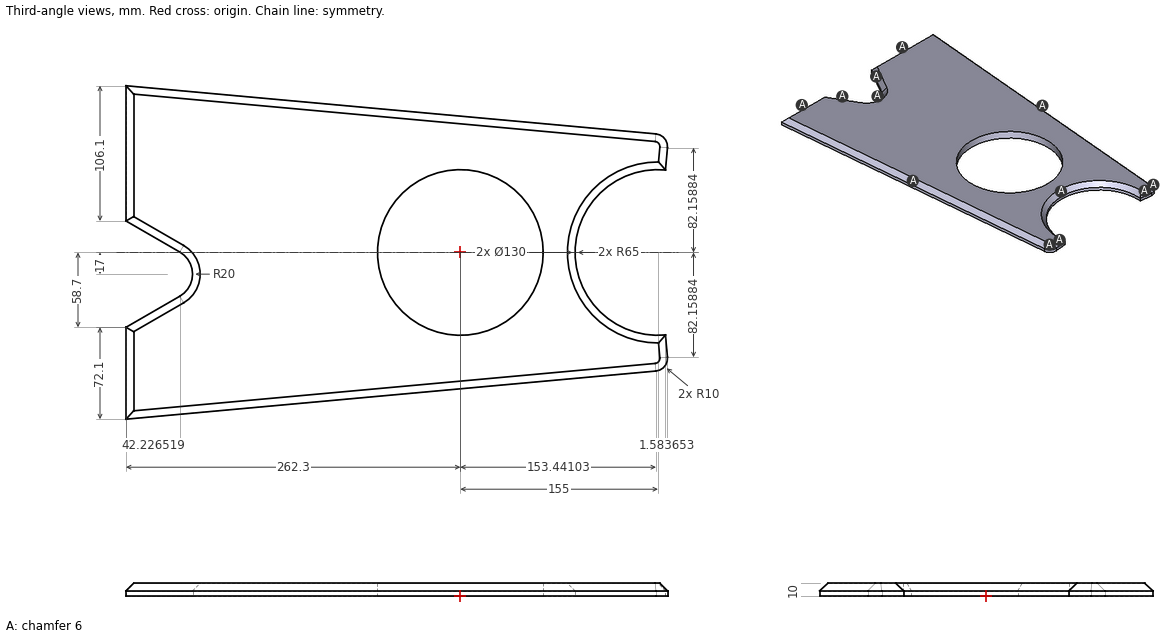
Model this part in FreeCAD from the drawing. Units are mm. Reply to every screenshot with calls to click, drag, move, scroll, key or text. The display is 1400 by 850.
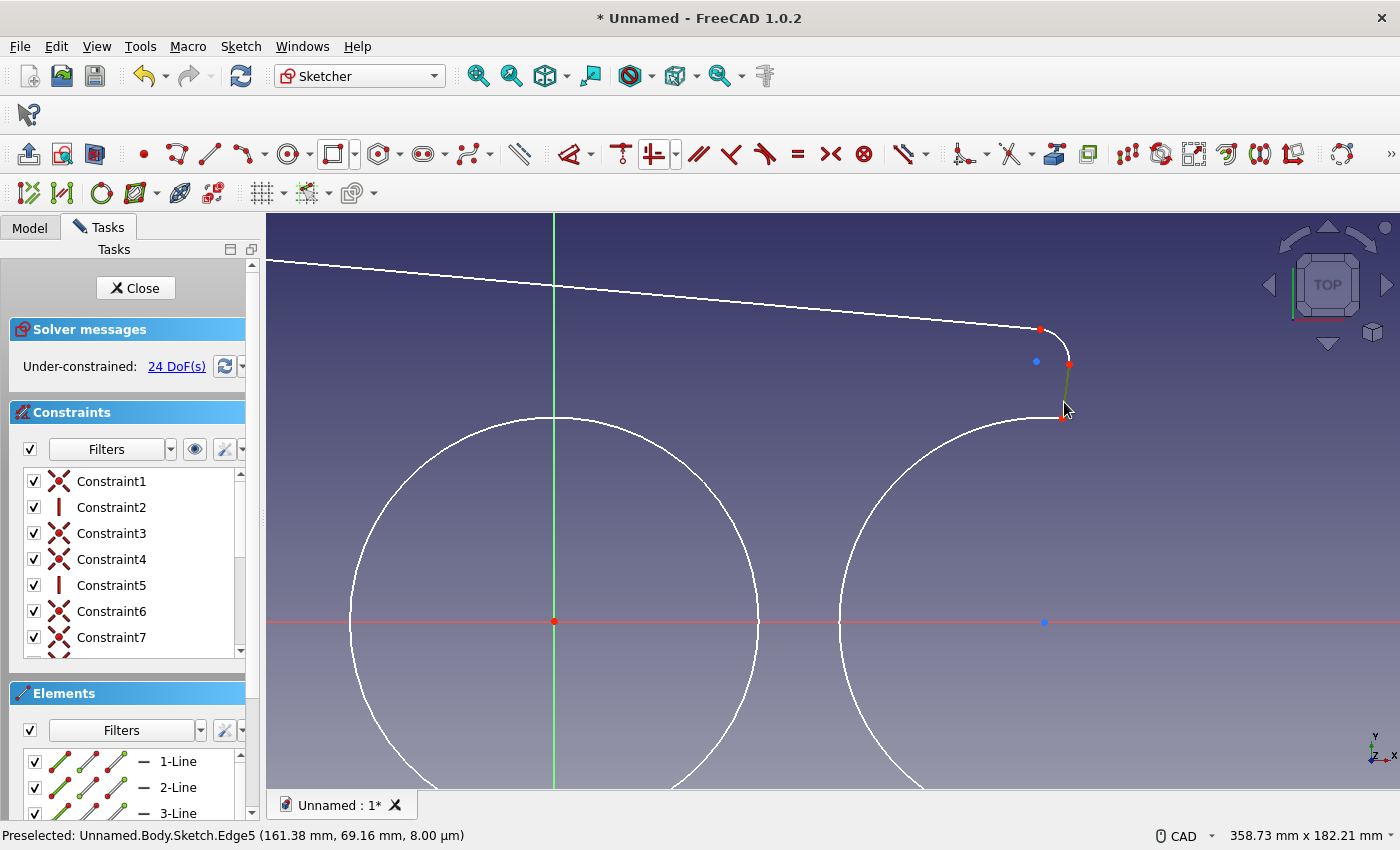
click(1067, 350)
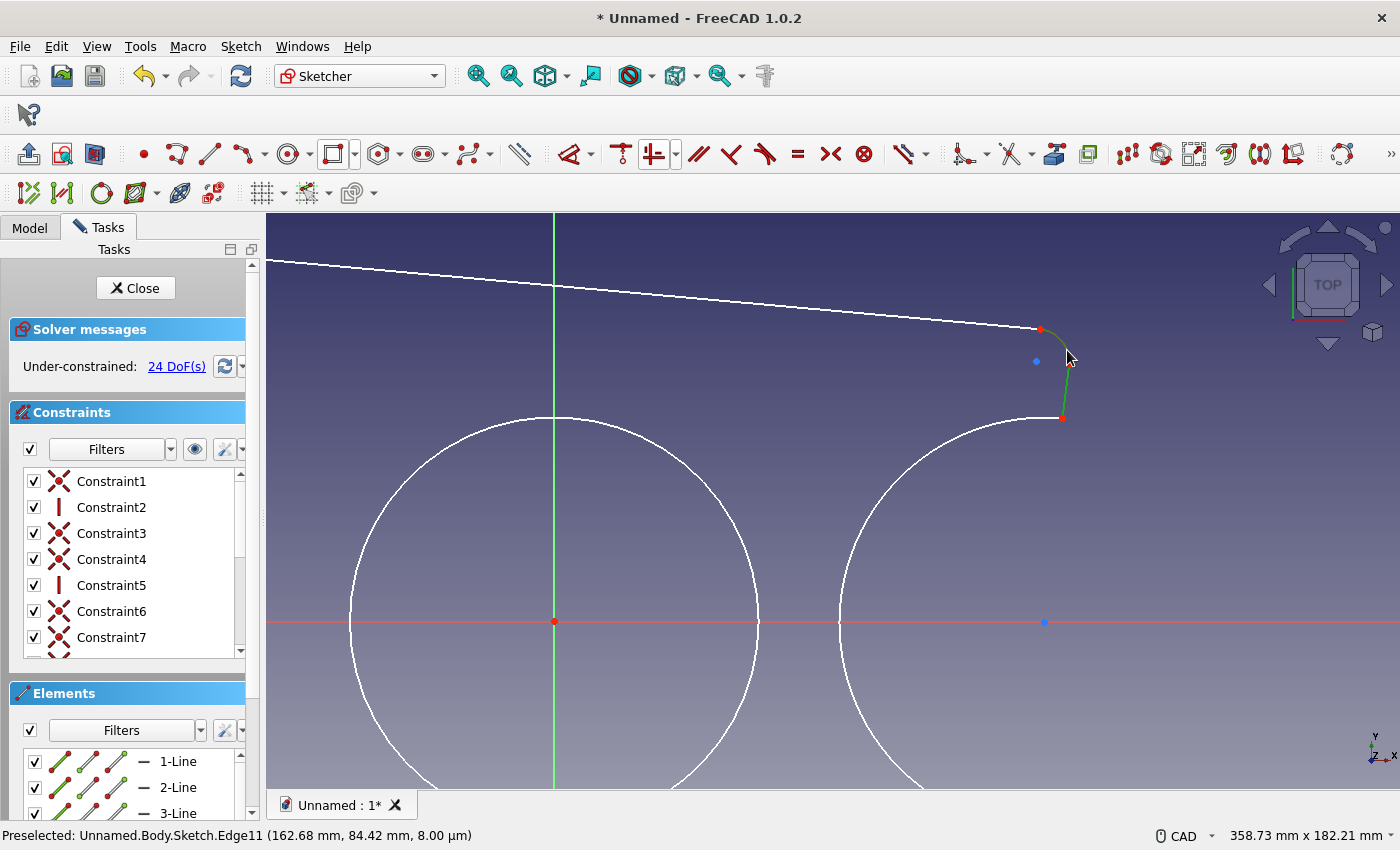
click(765, 154)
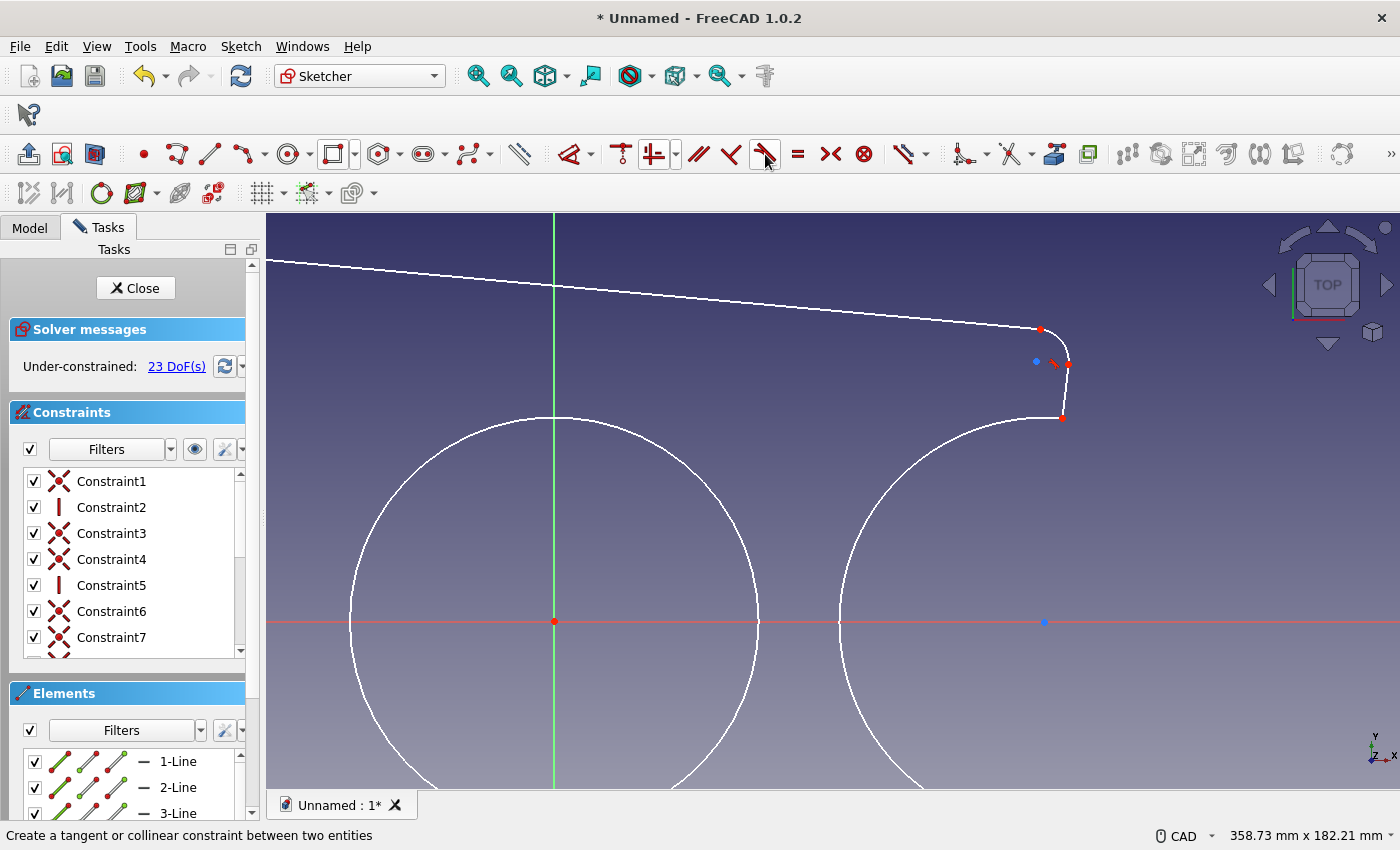
click(646, 294)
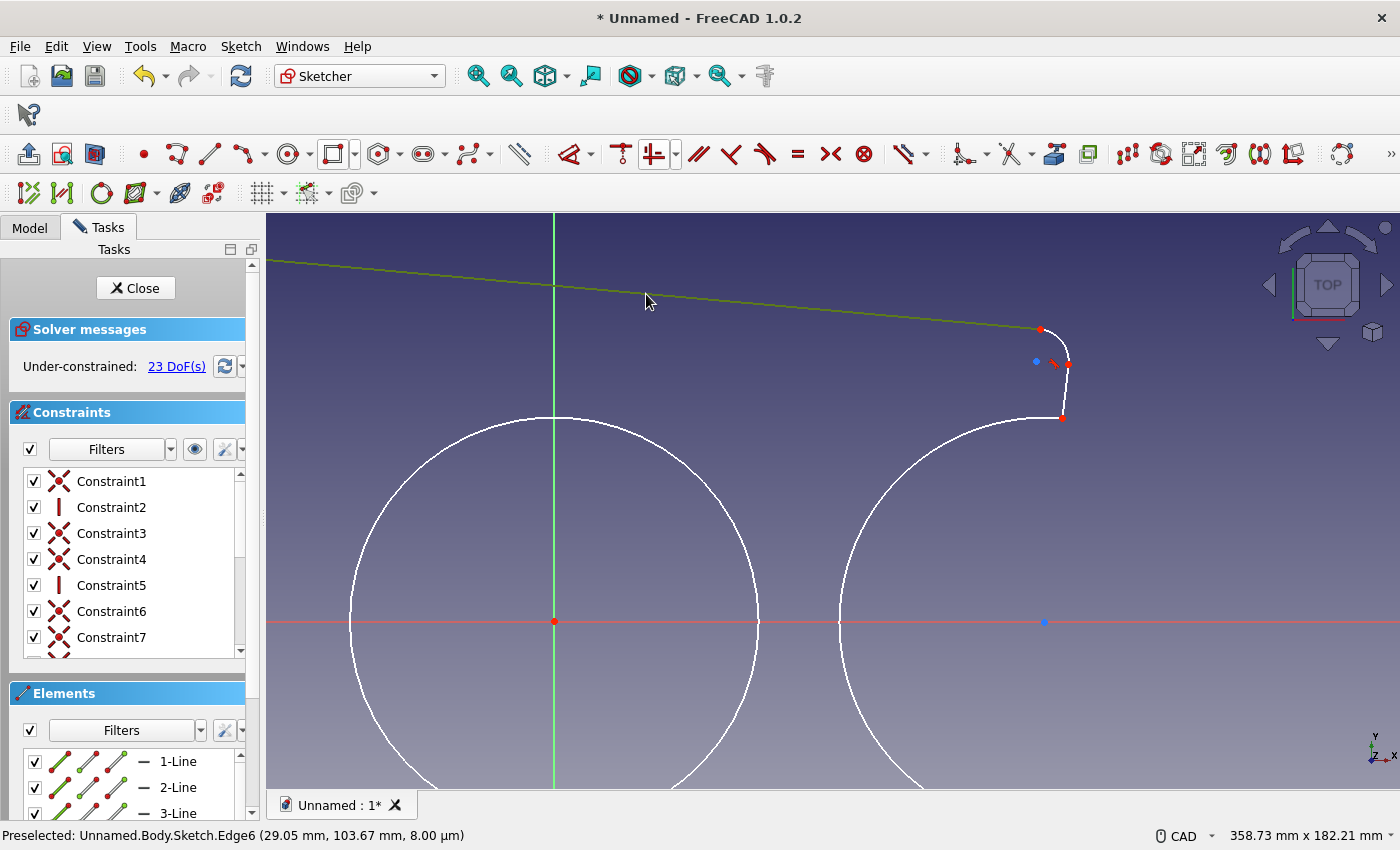
click(1067, 350)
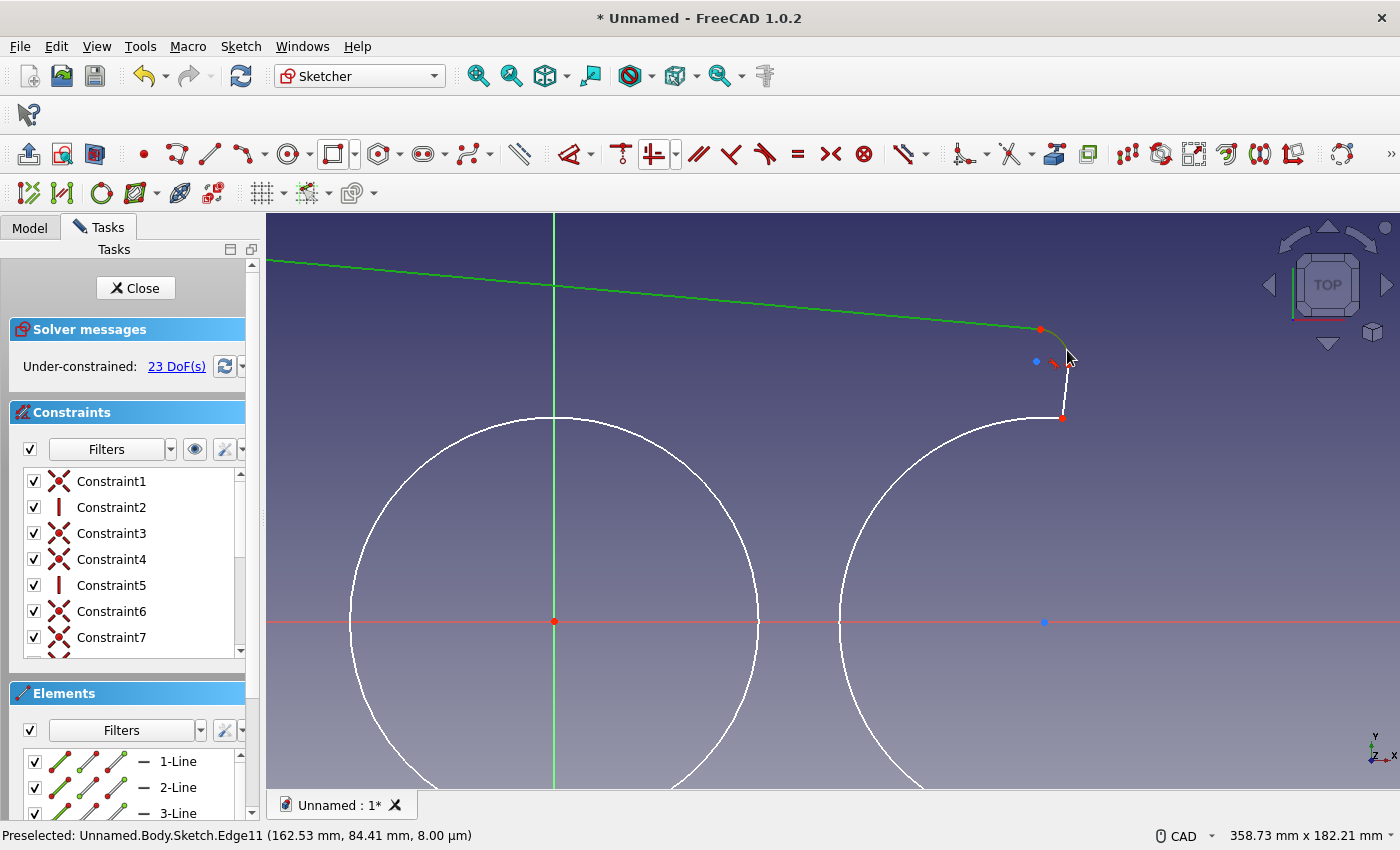
click(765, 154)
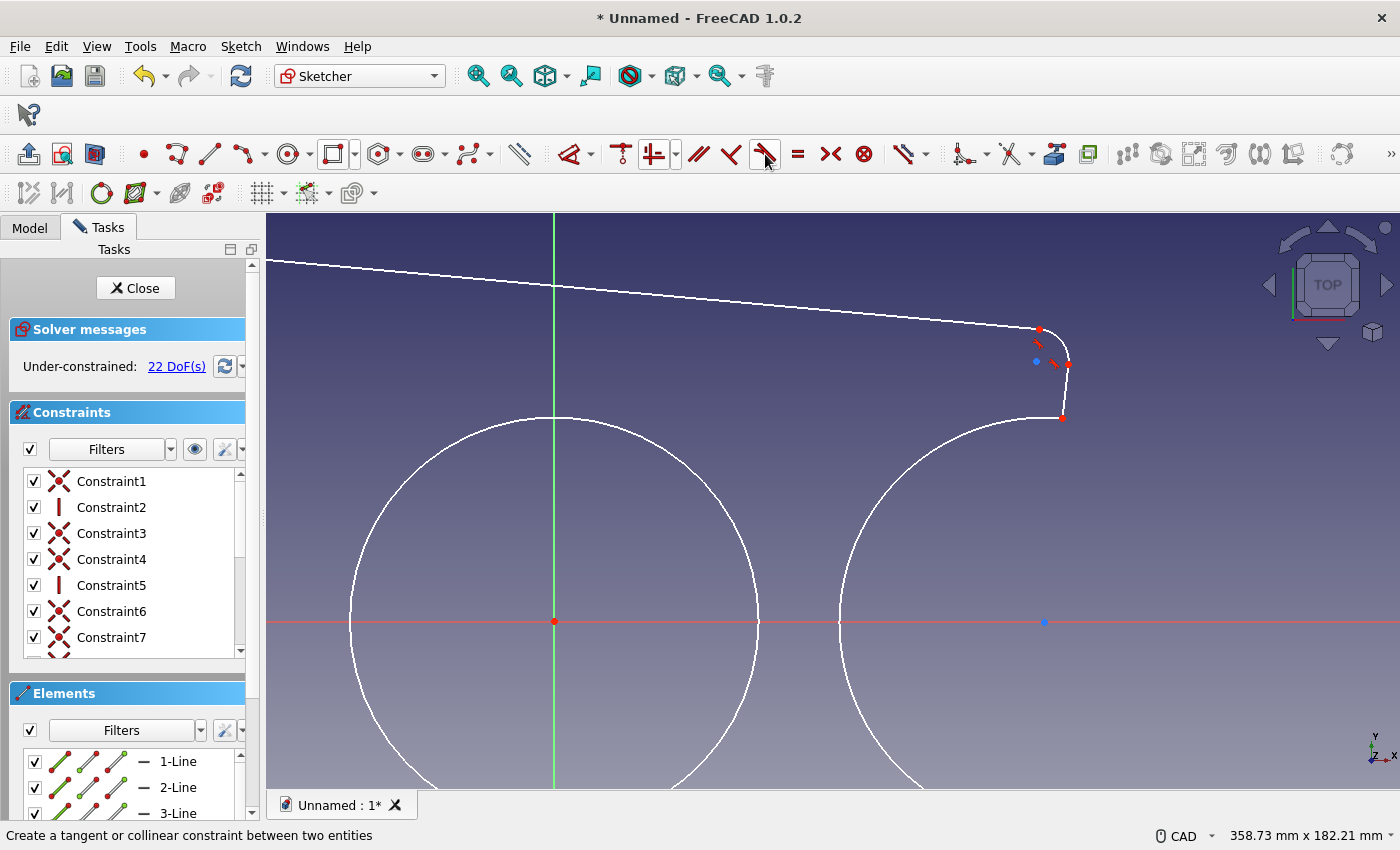
scroll(1065, 403, down, 4)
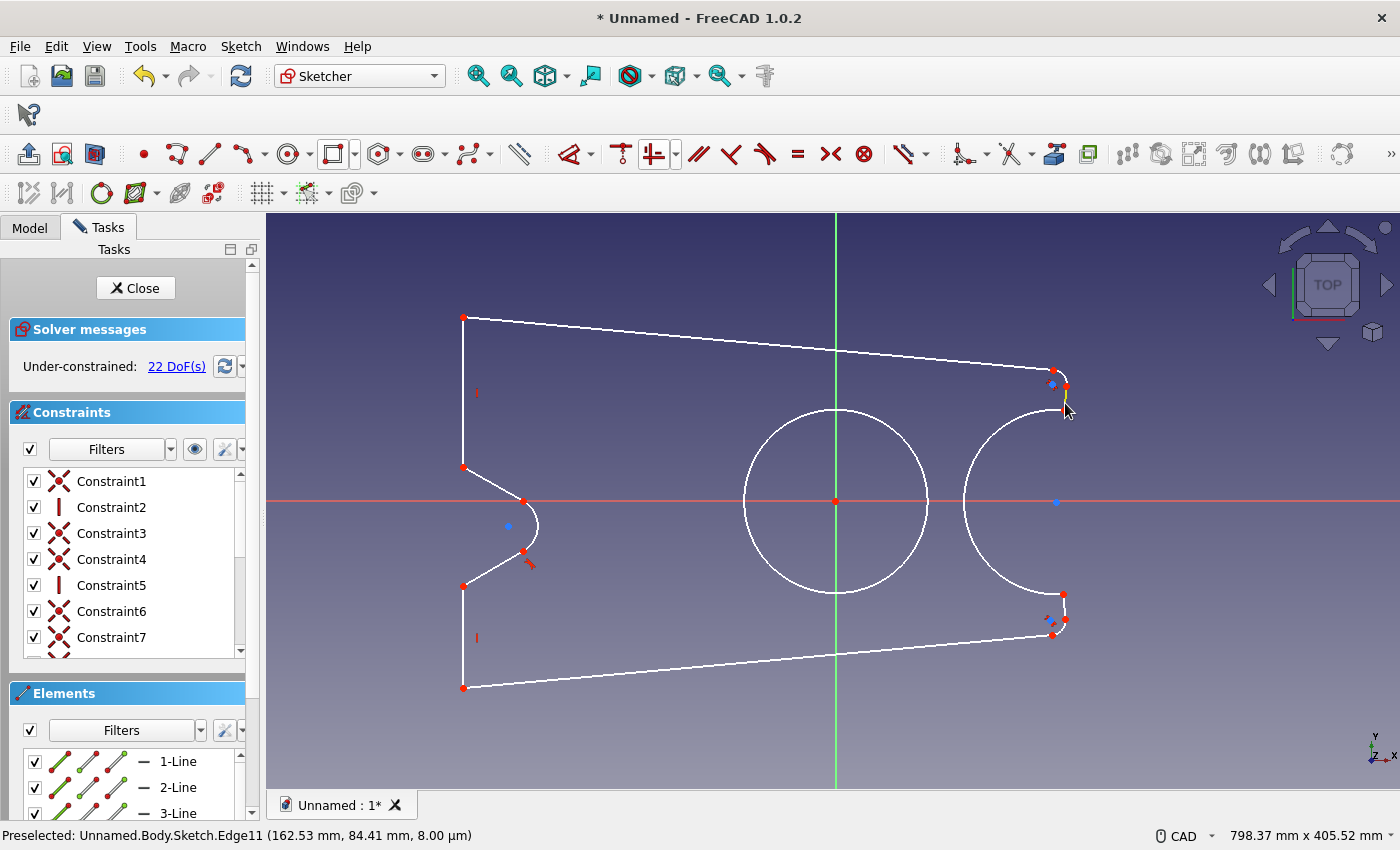
click(481, 477)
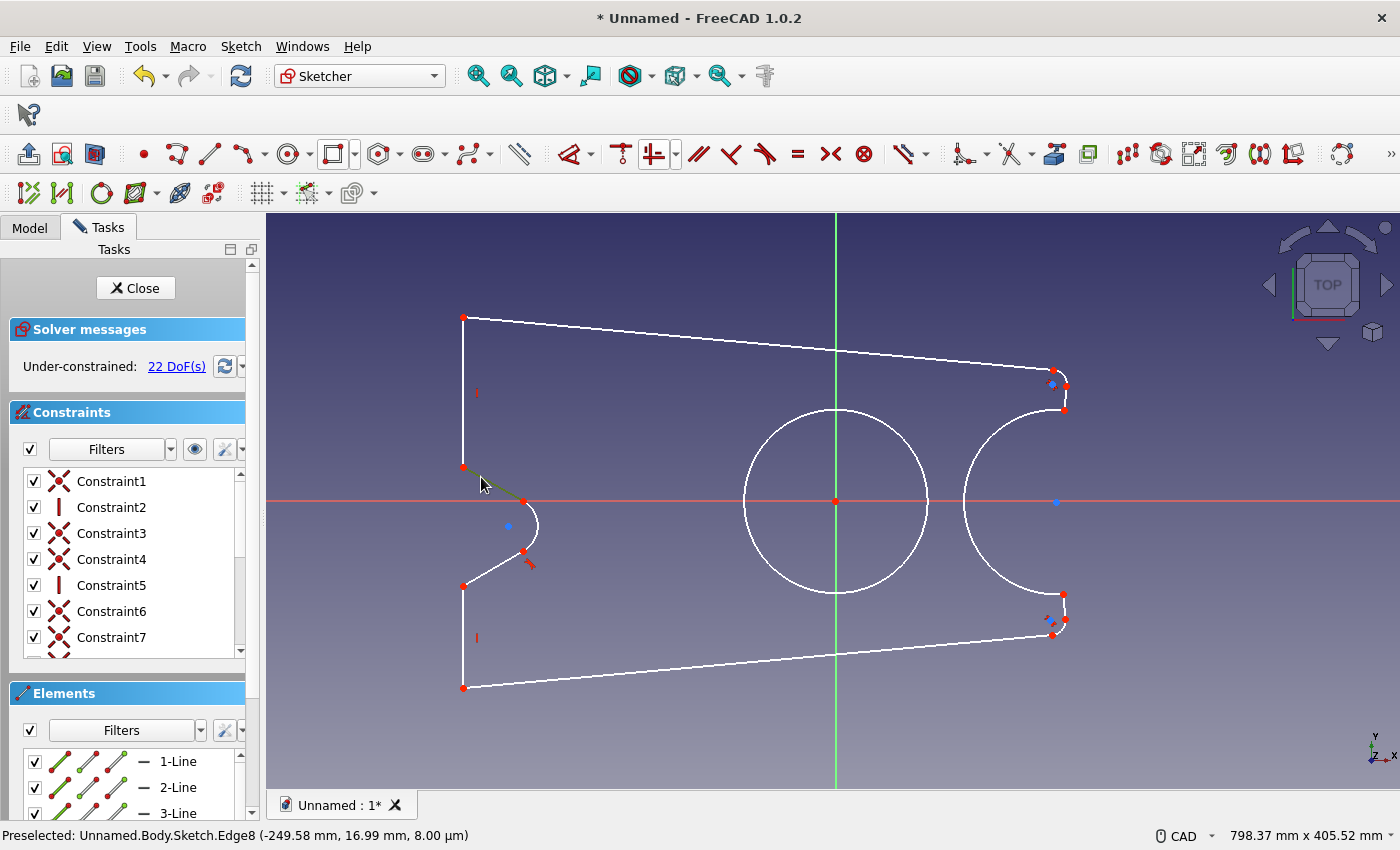
click(535, 538)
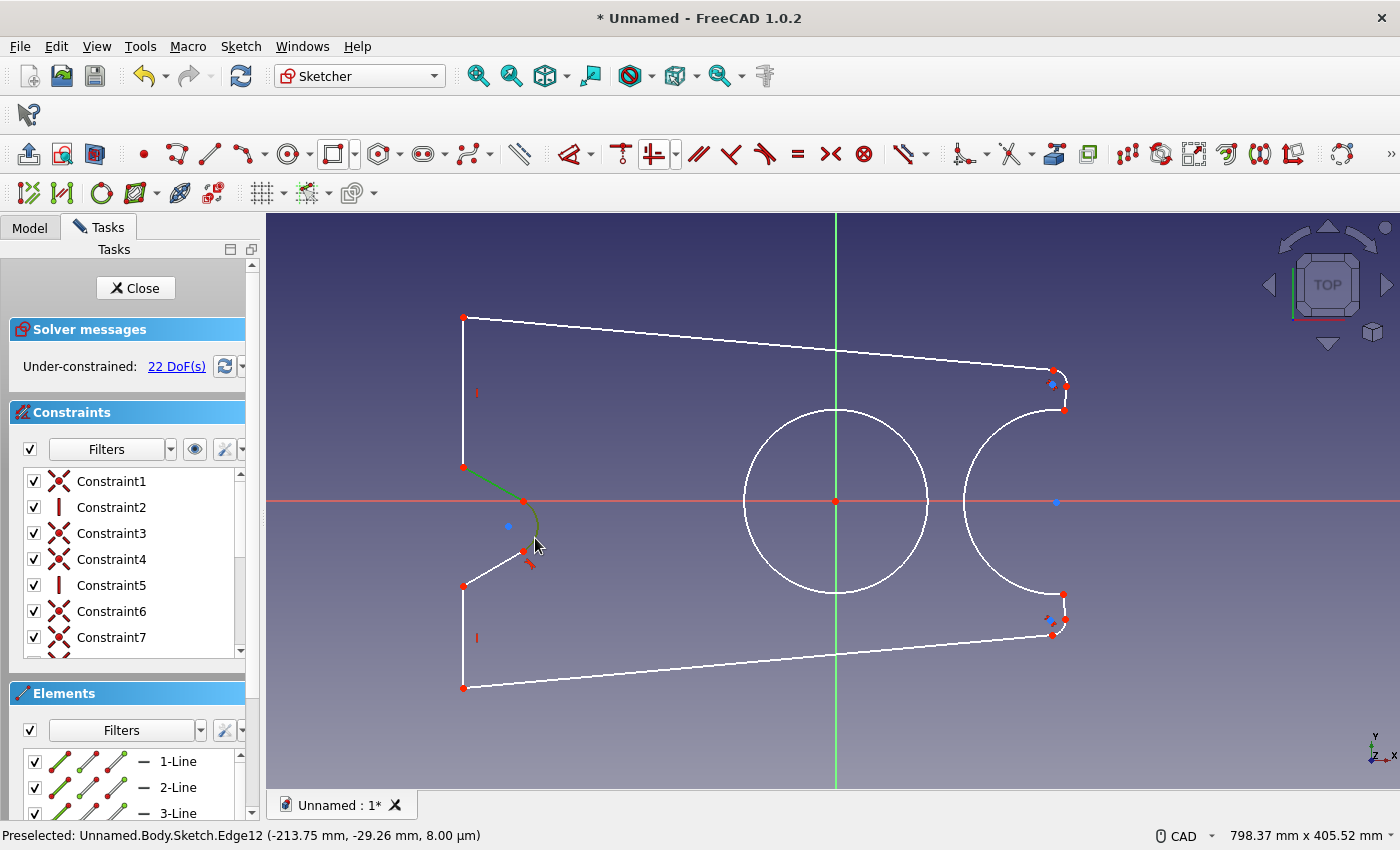
click(765, 154)